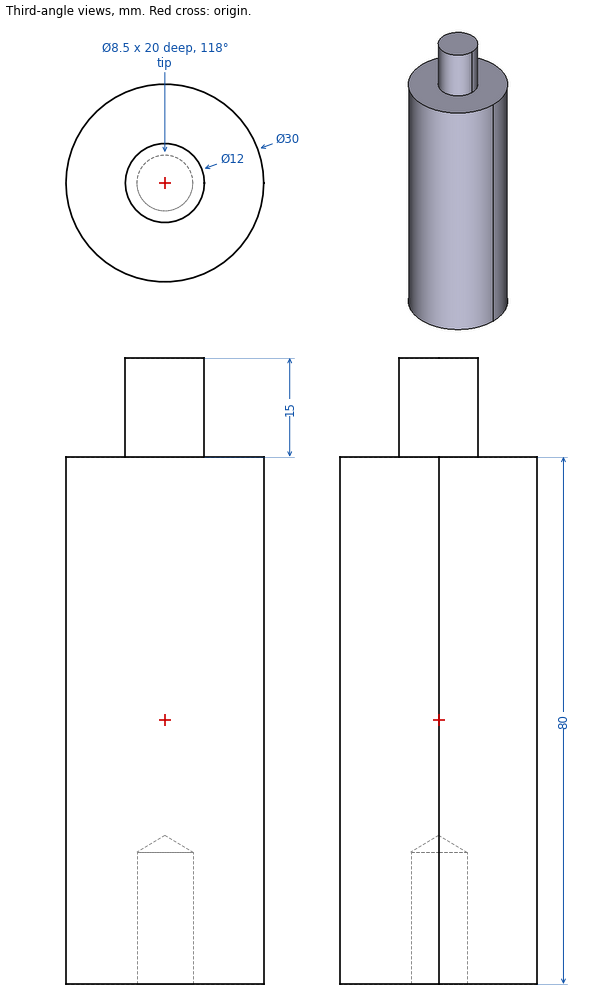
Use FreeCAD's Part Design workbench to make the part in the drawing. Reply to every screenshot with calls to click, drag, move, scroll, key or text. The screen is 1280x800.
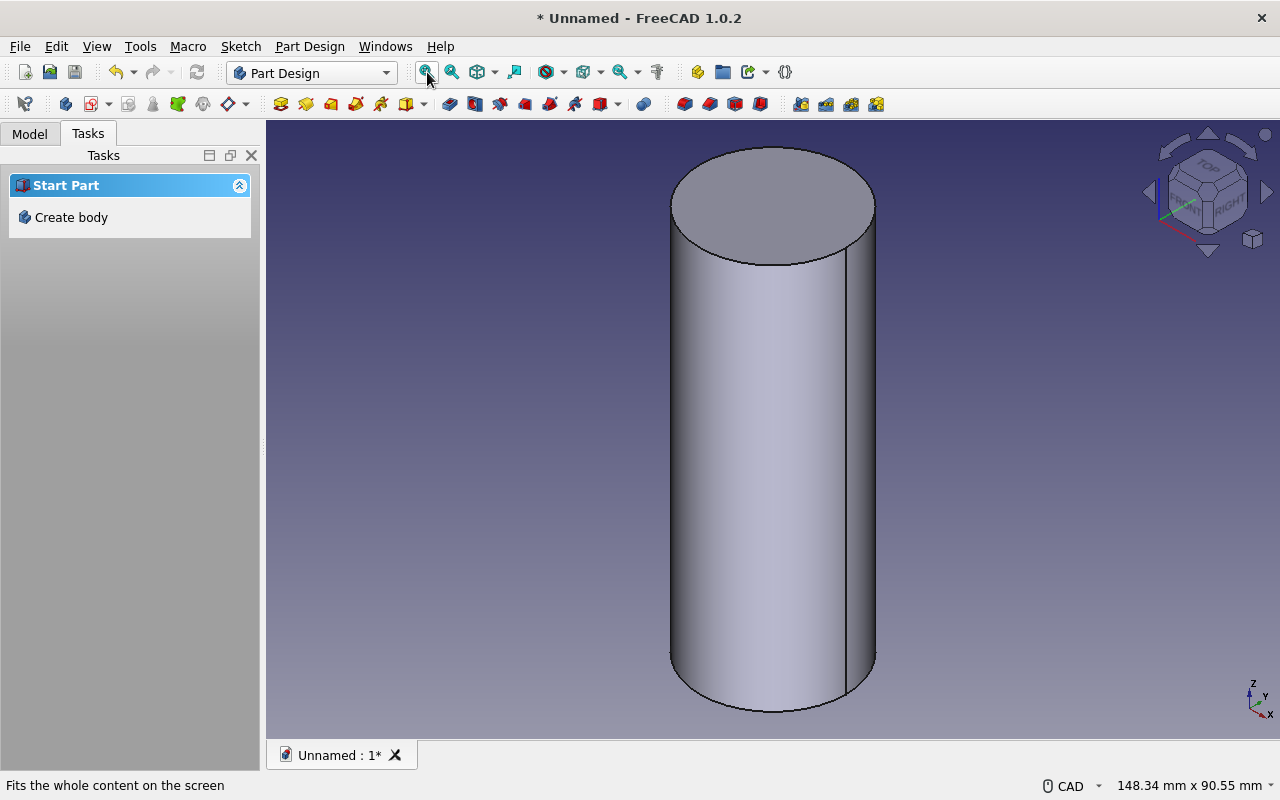
click(773, 205)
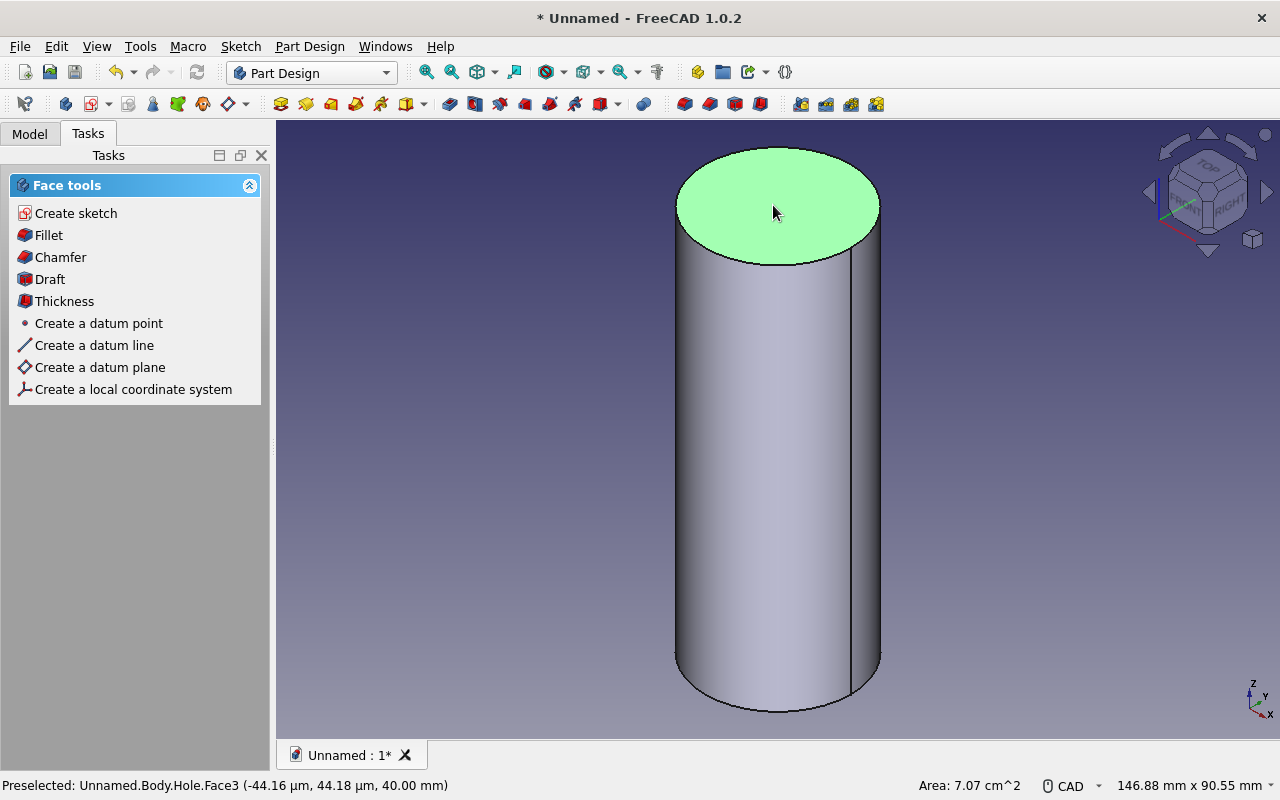
click(90, 104)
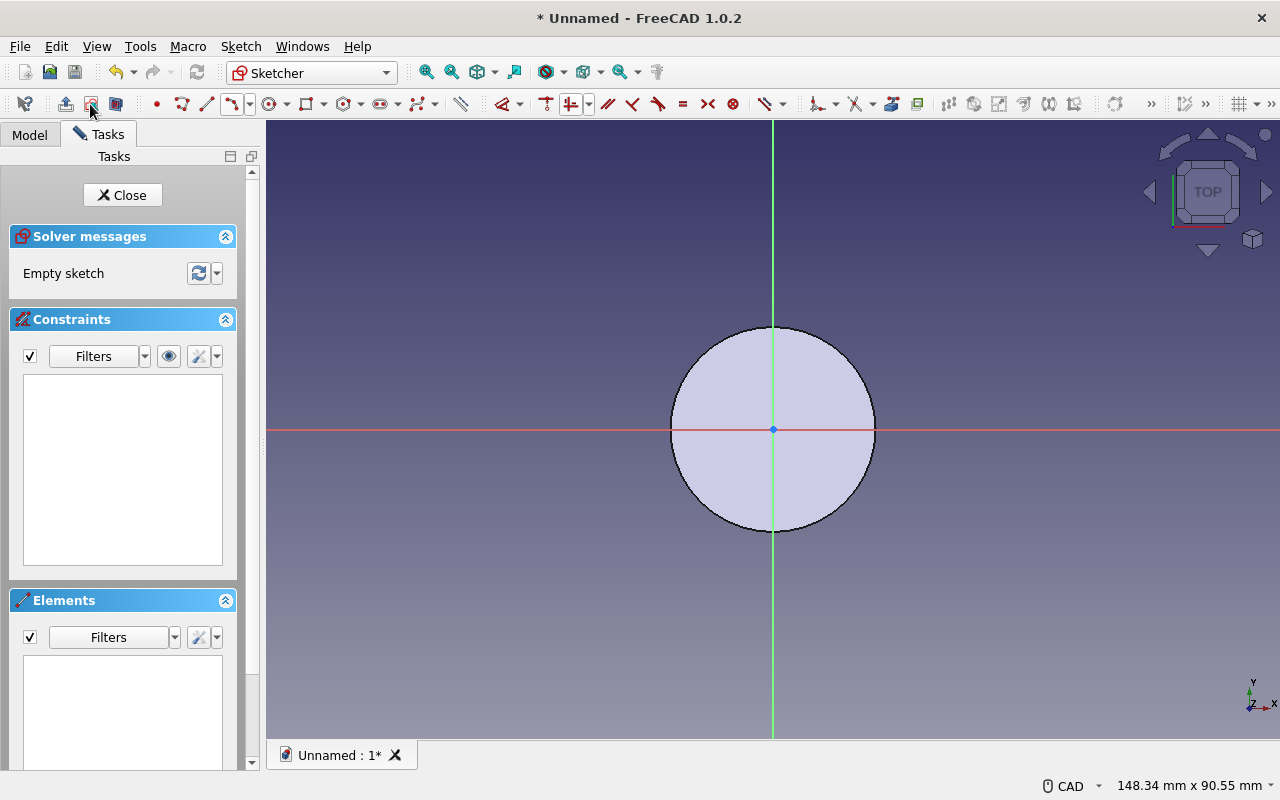
scroll(790, 430, up, 8)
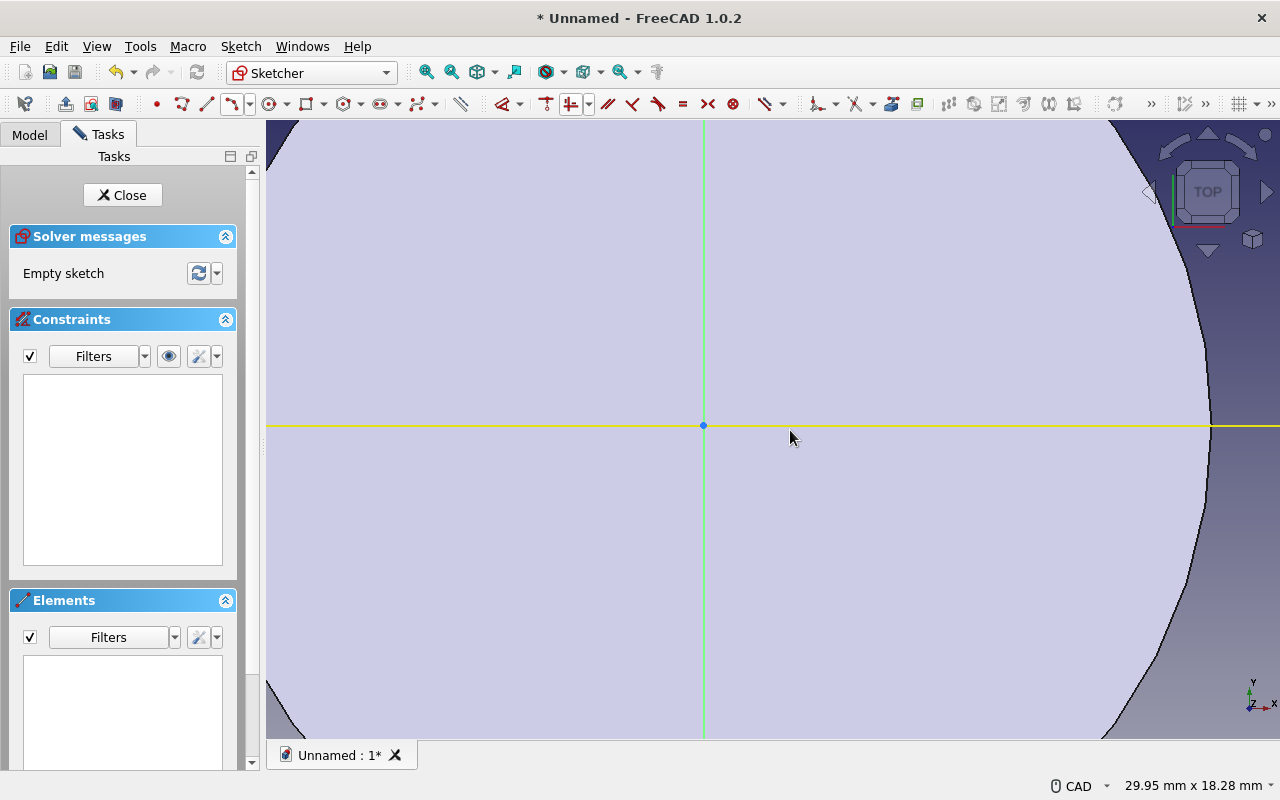
click(268, 104)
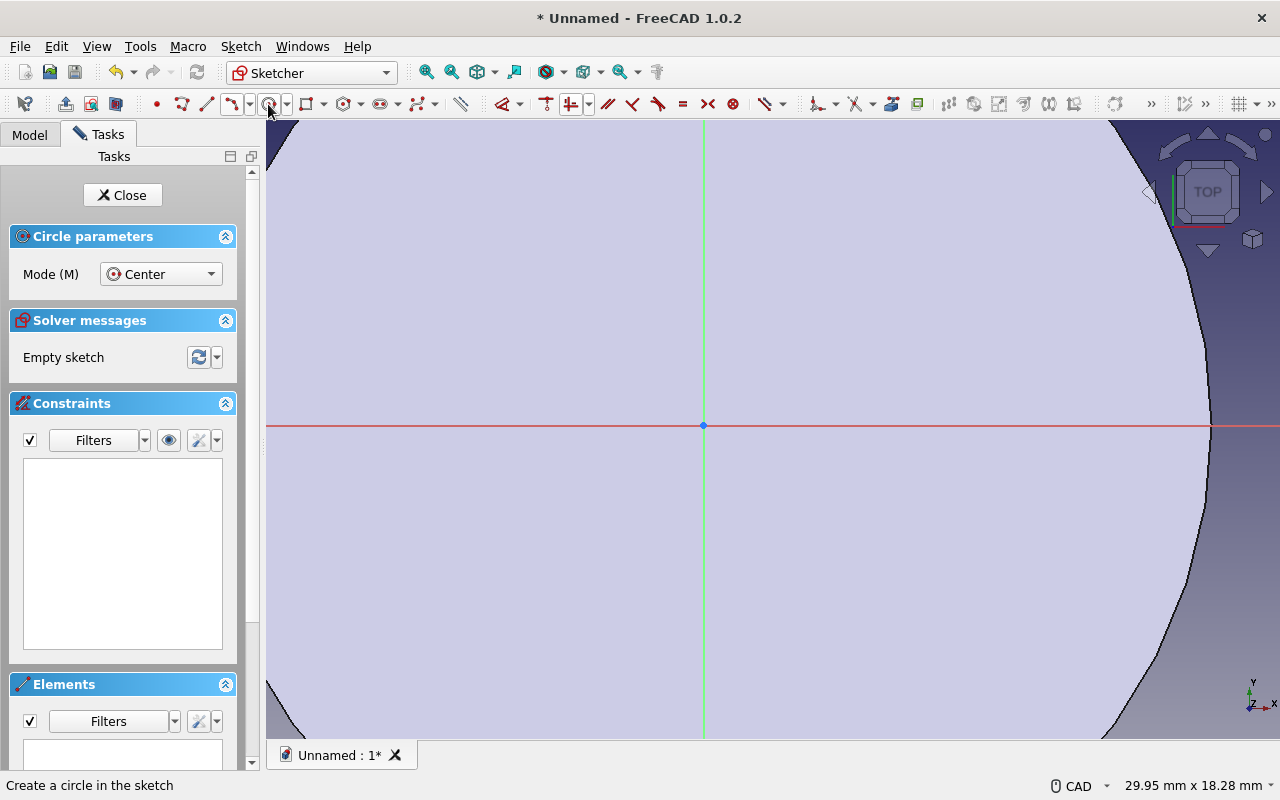
click(704, 426)
move(847, 282)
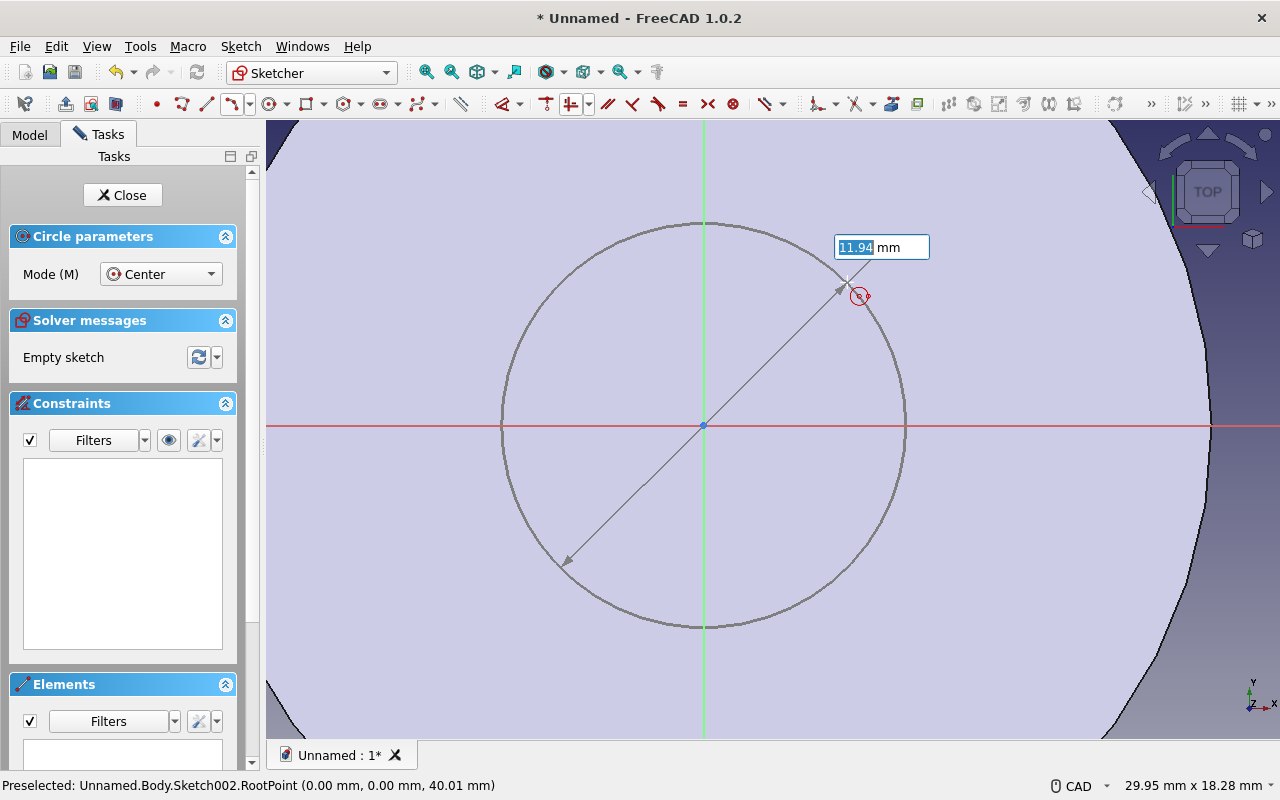
text(12)
key(Return)
key(Escape)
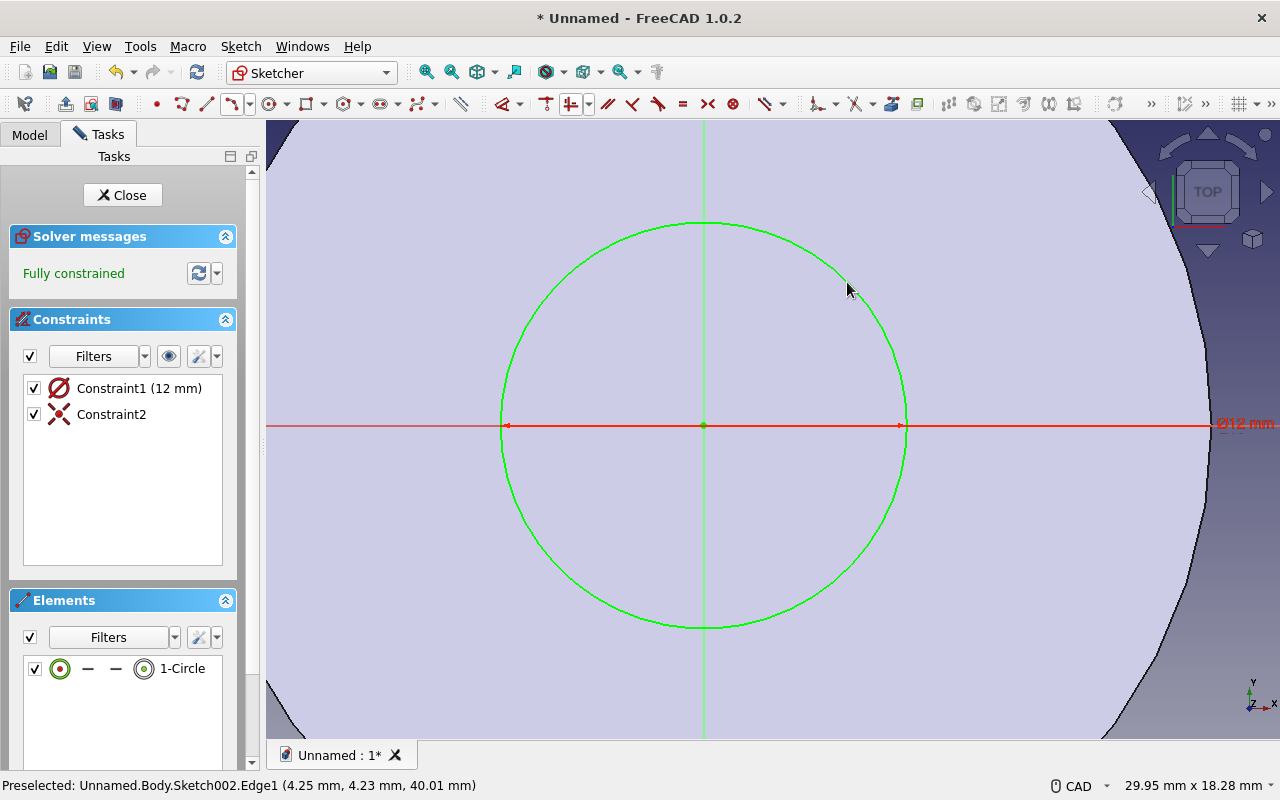
click(123, 195)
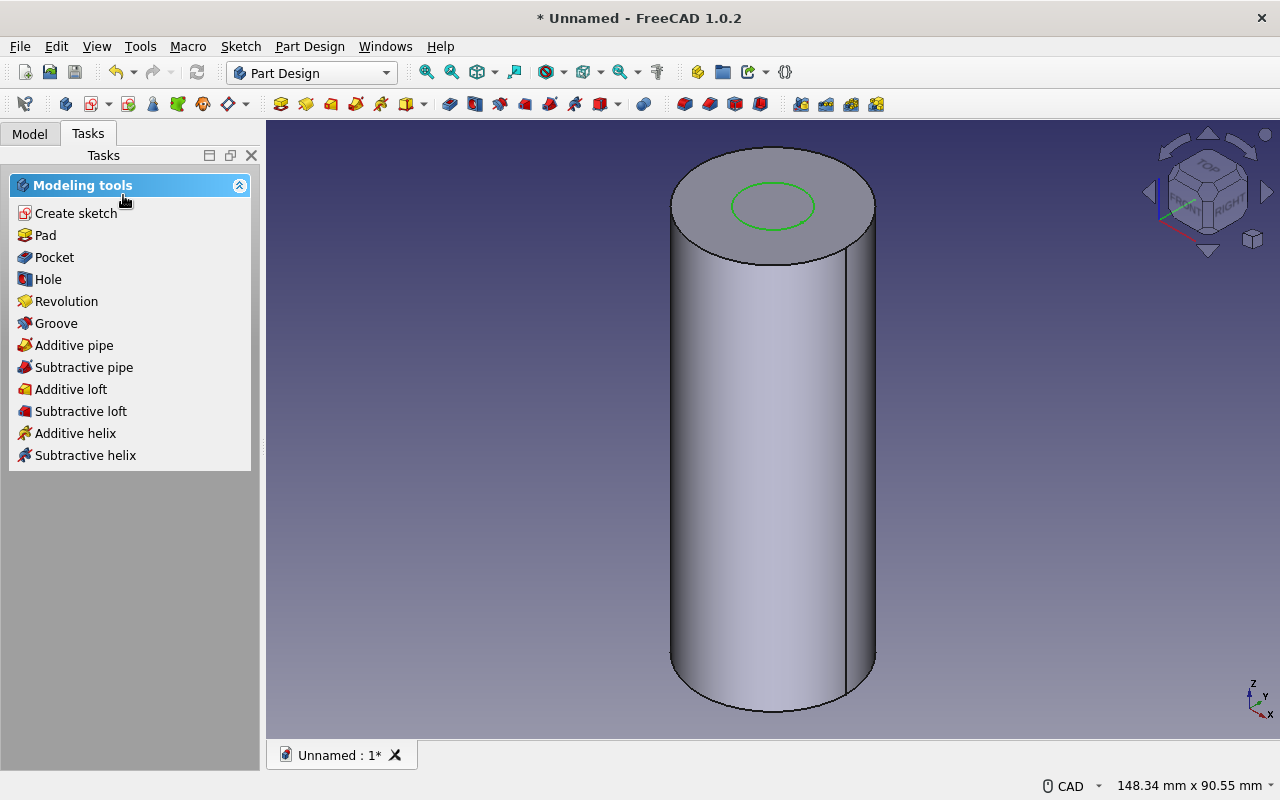
click(281, 104)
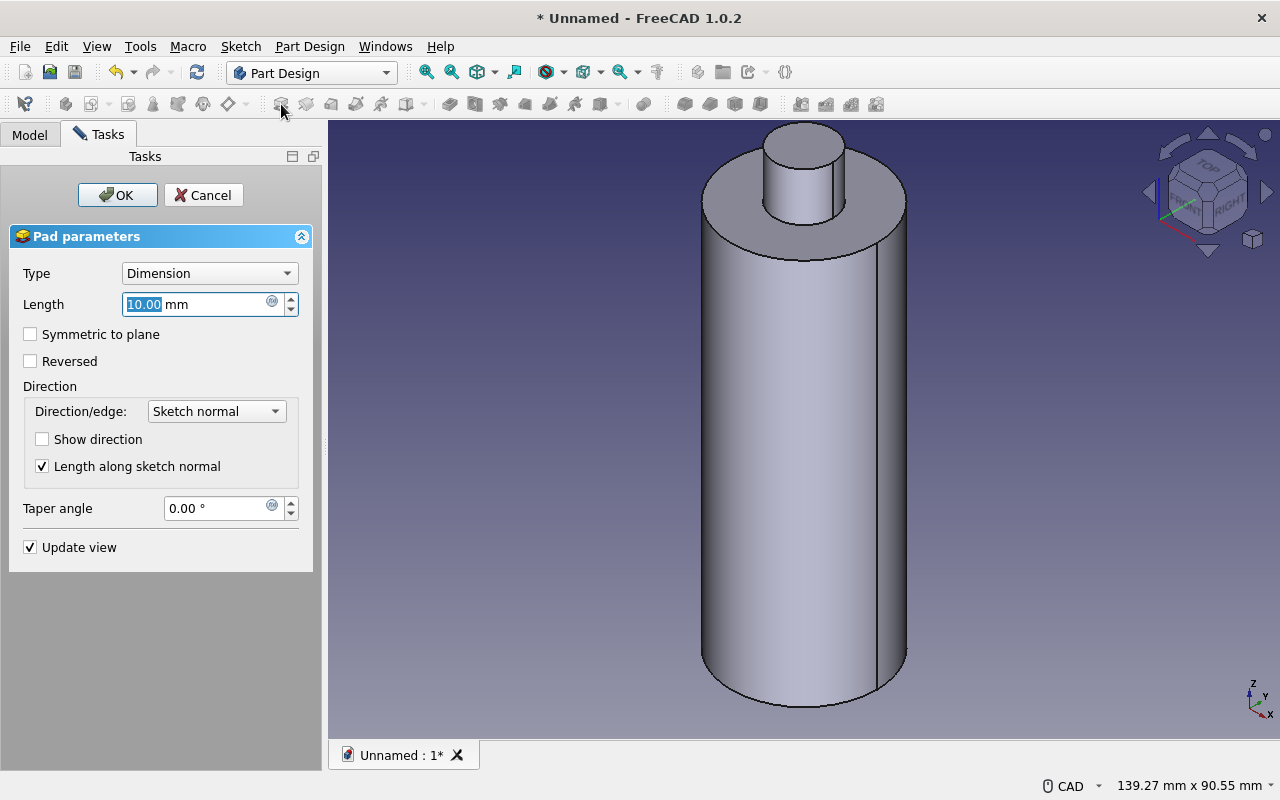
text(15)
key(Tab)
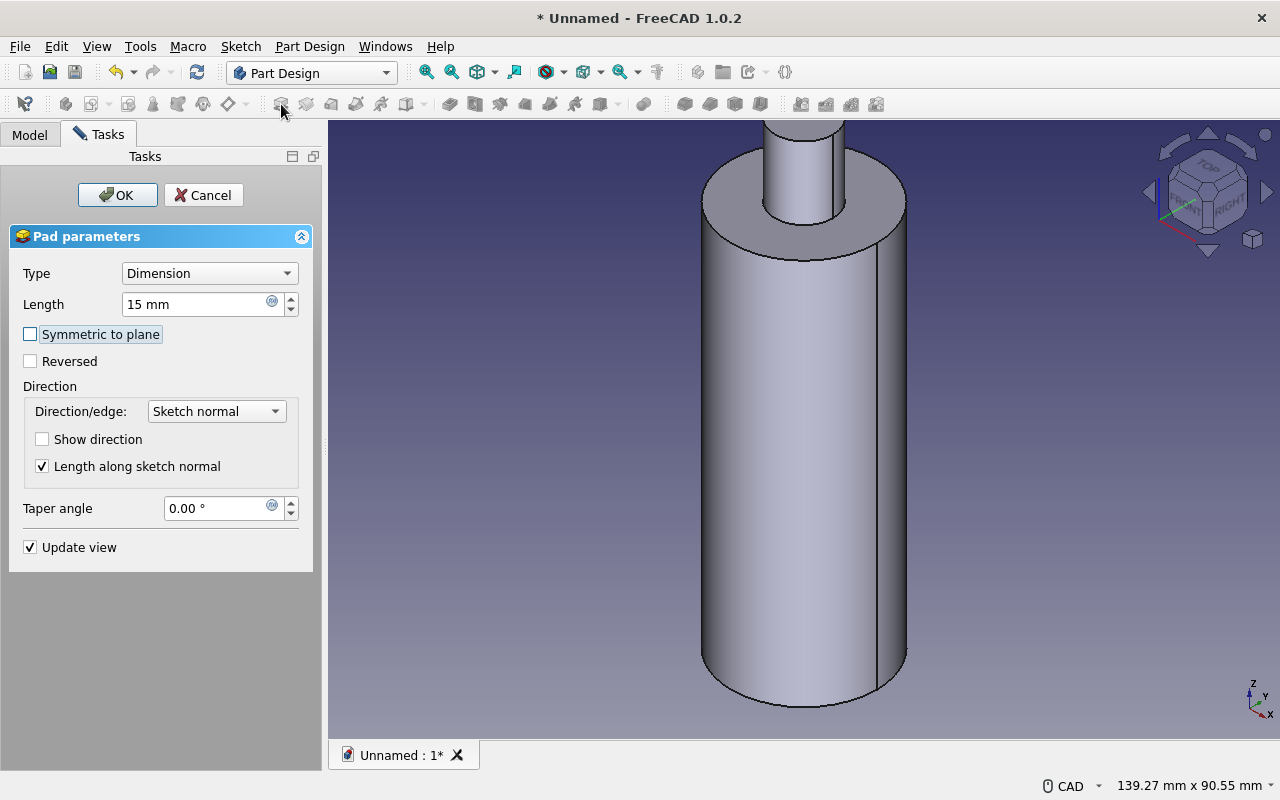
click(118, 195)